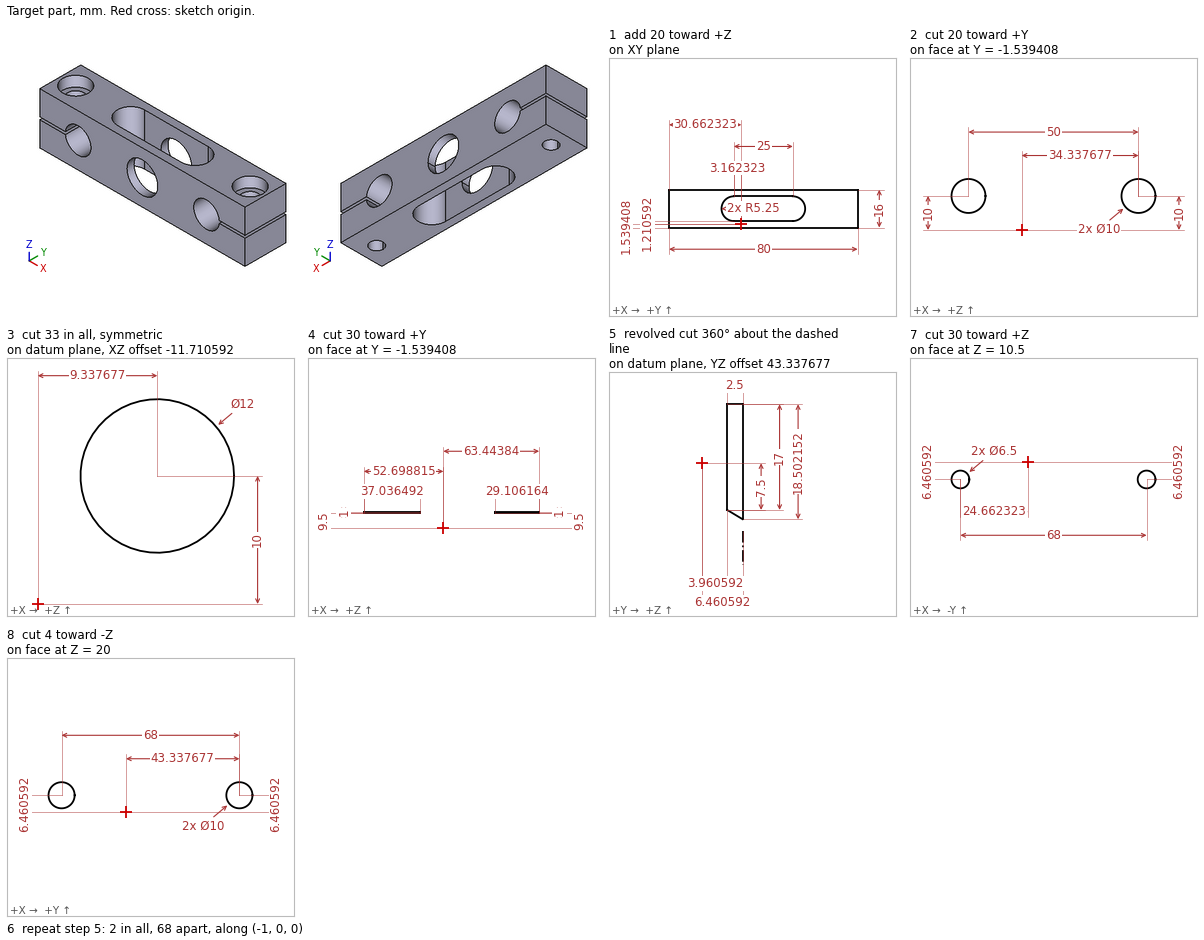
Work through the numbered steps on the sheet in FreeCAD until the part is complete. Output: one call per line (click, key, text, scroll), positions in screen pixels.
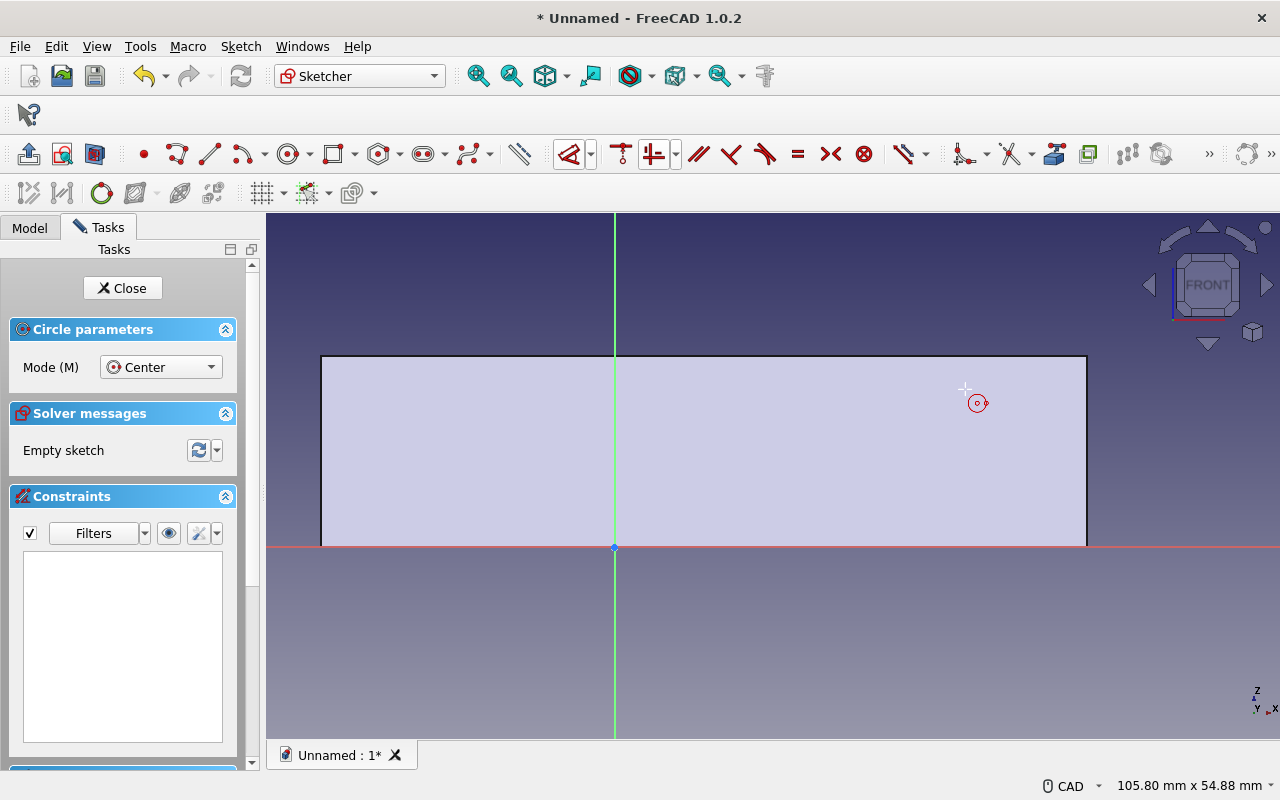
click(944, 451)
move(978, 418)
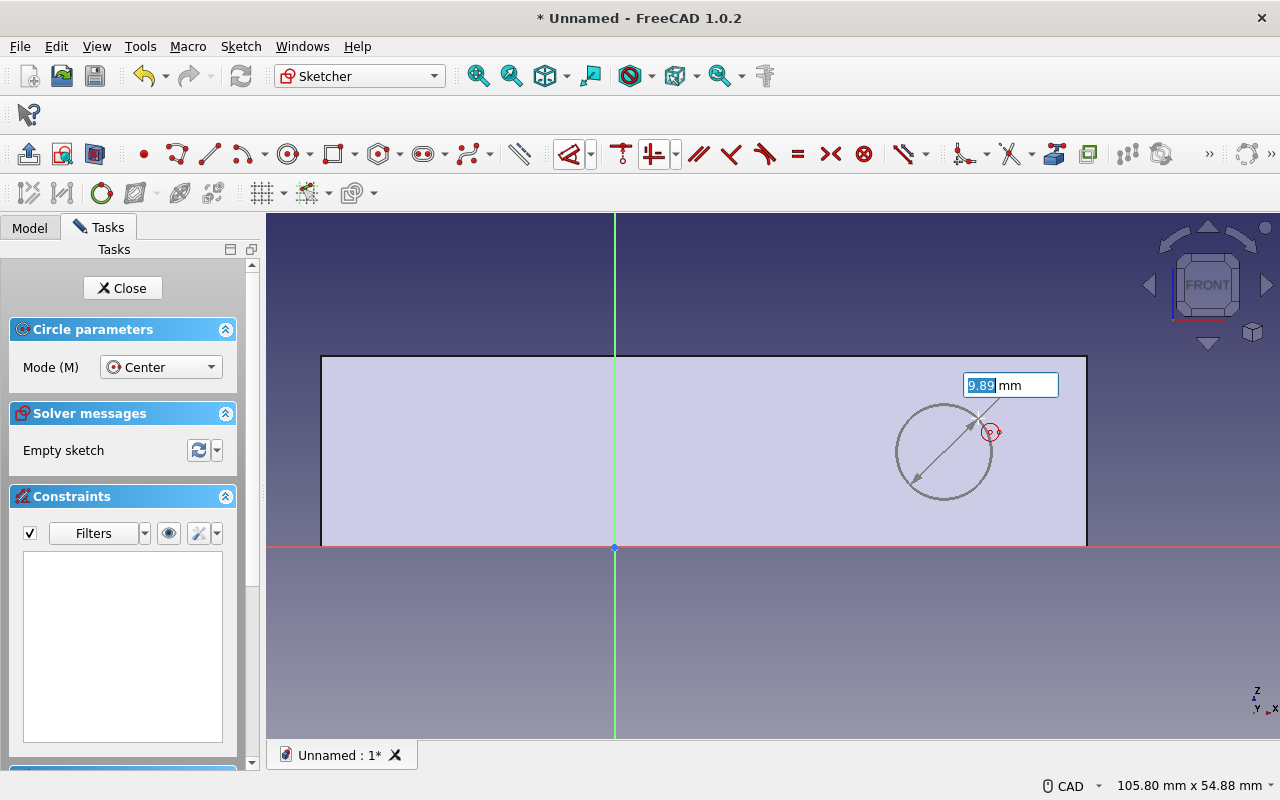
text(10)
key(Return)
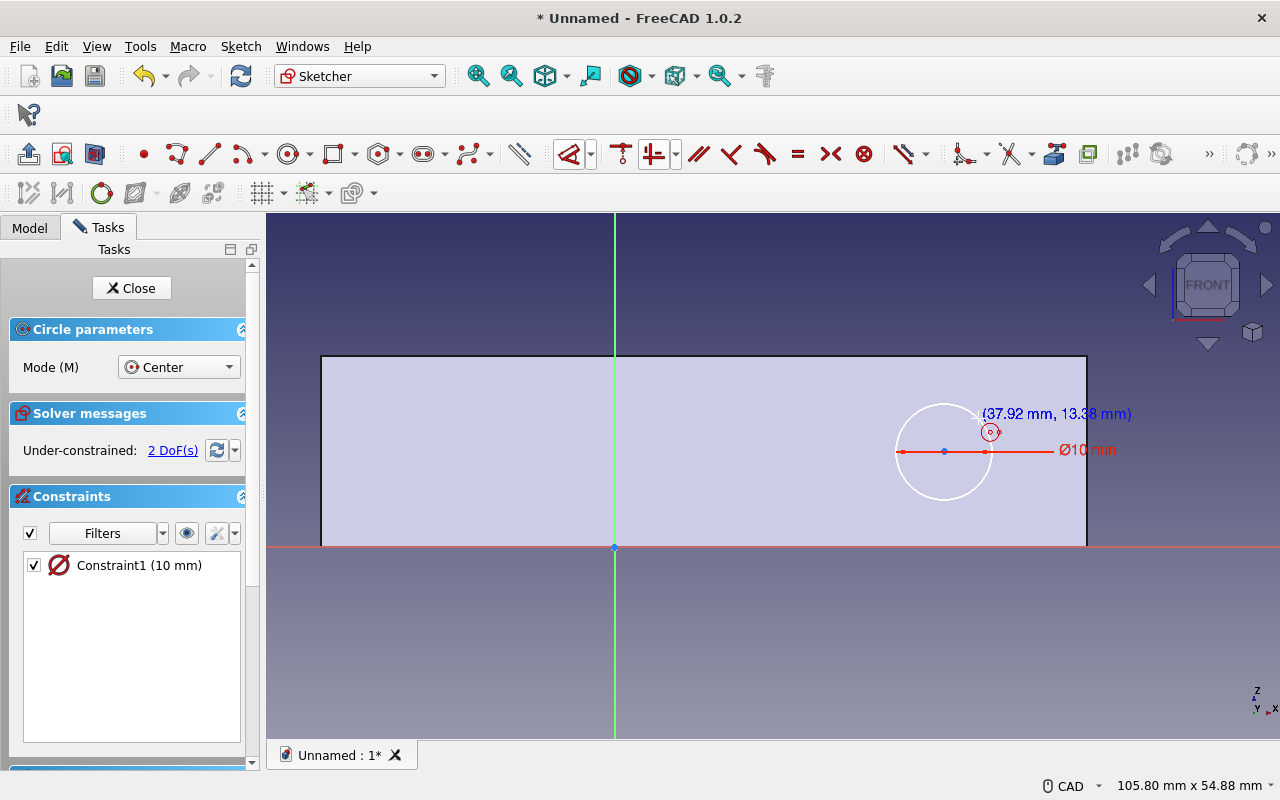
click(464, 451)
move(498, 418)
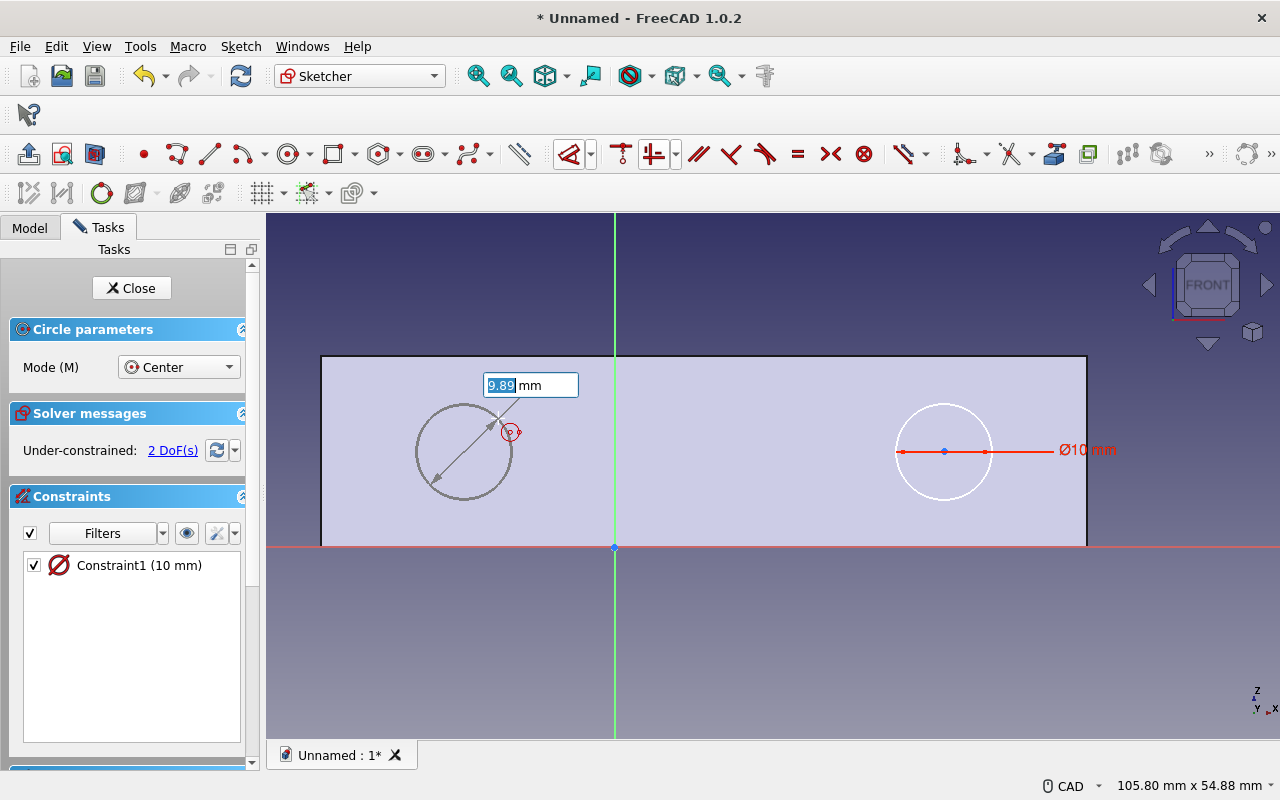
text(10)
key(Return)
key(Escape)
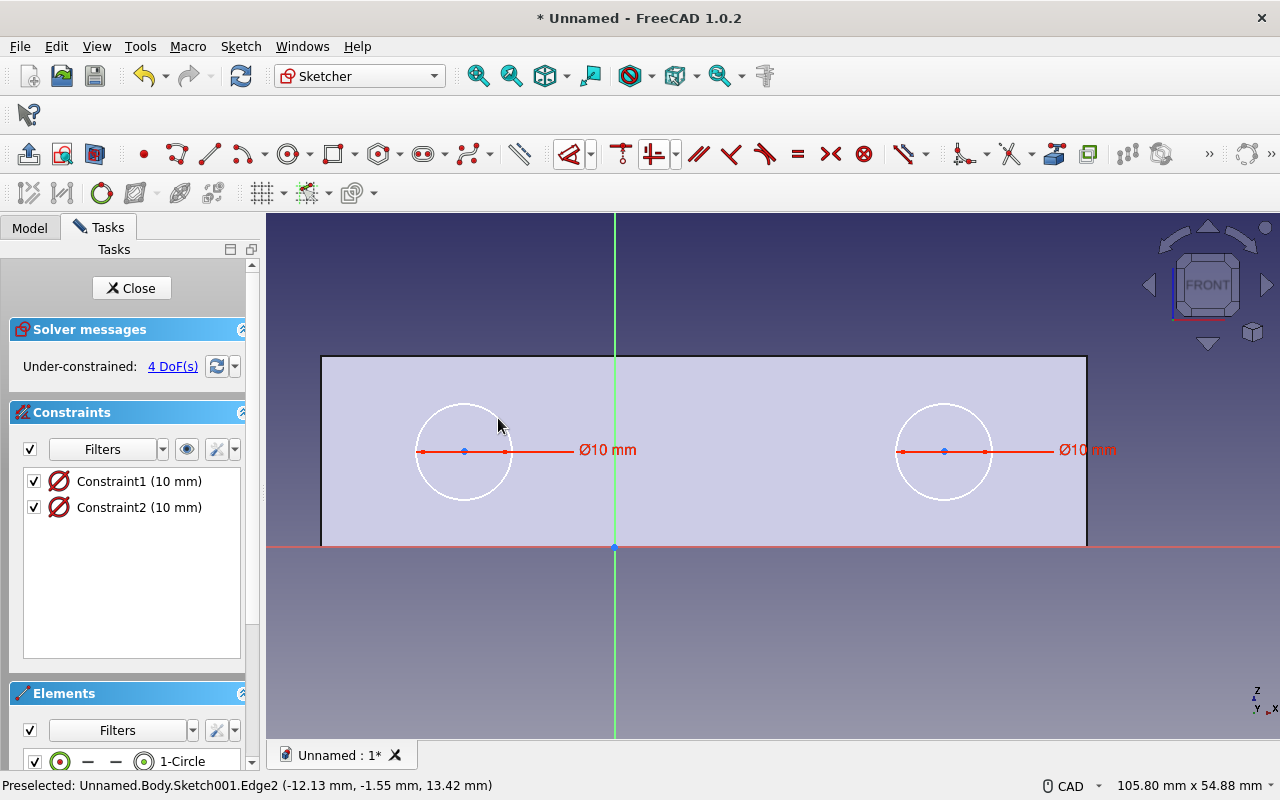
click(944, 452)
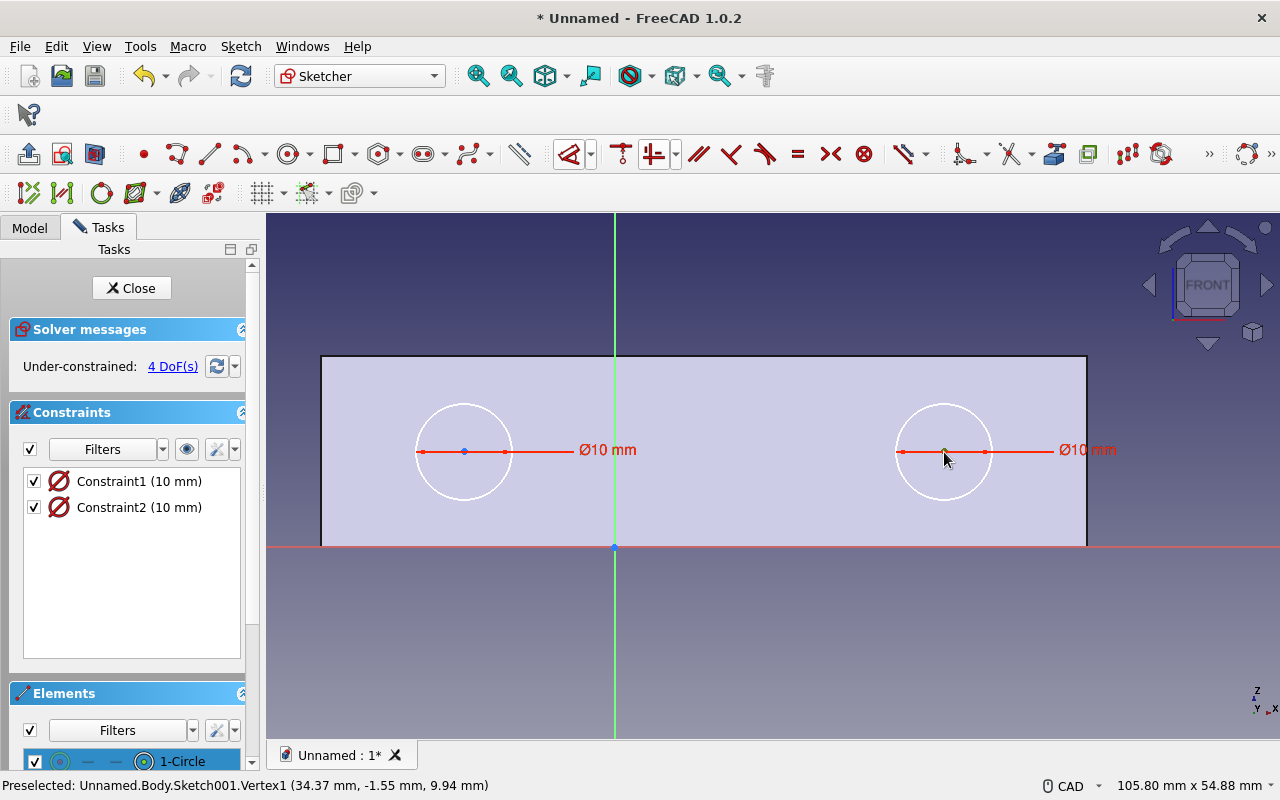
click(590, 154)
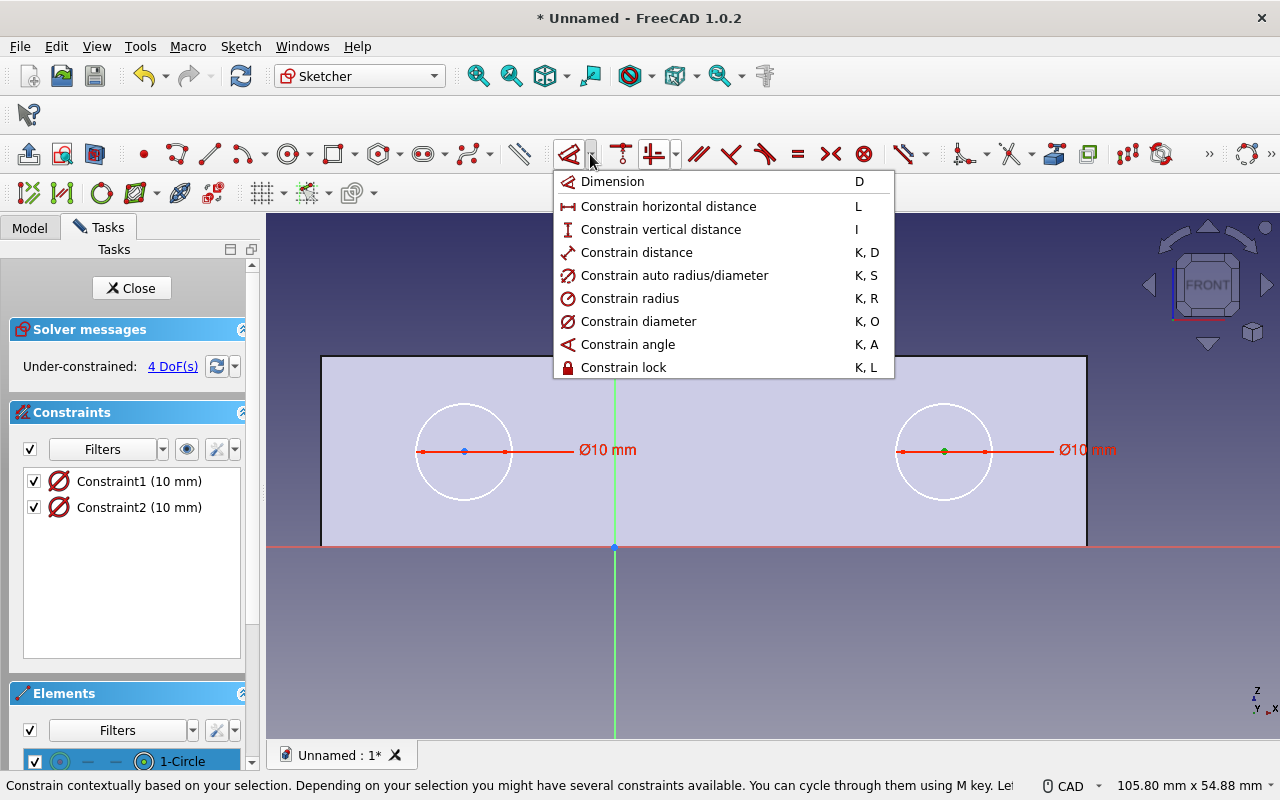
click(724, 230)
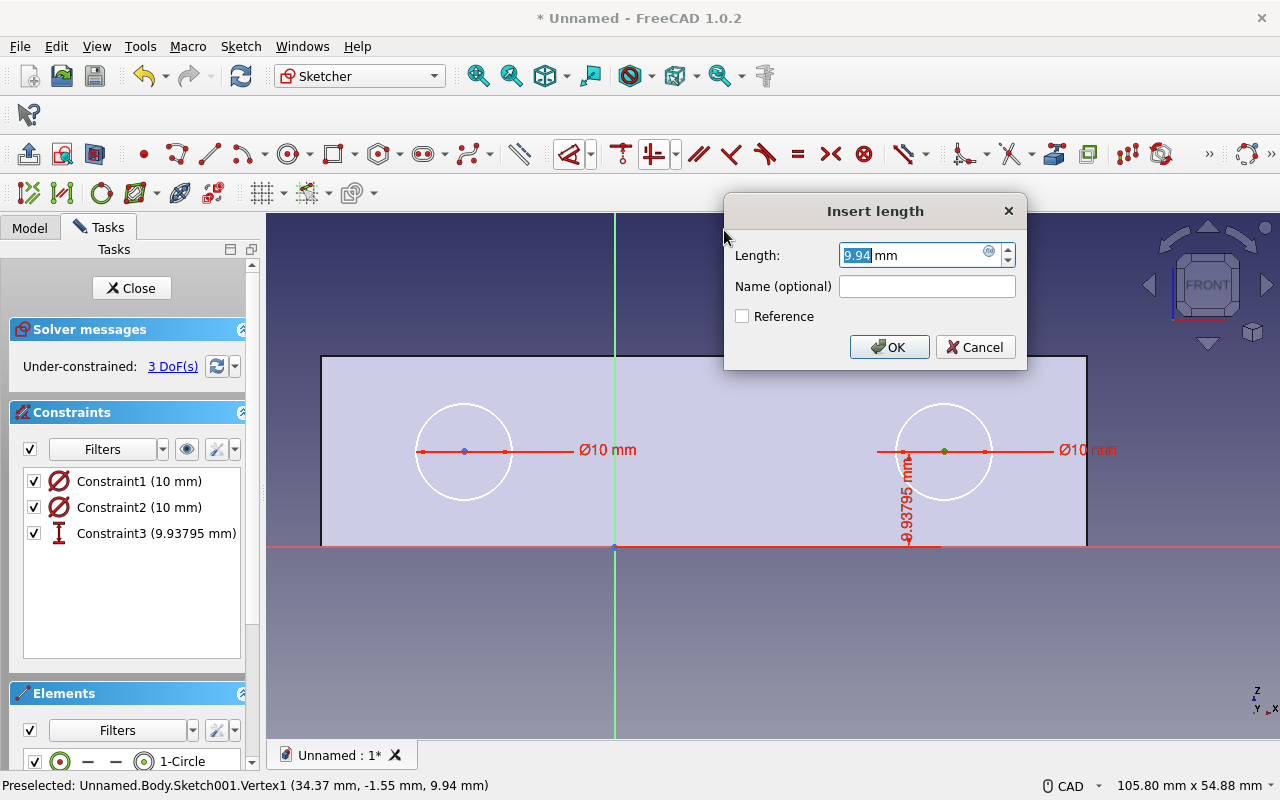
text(10)
key(Return)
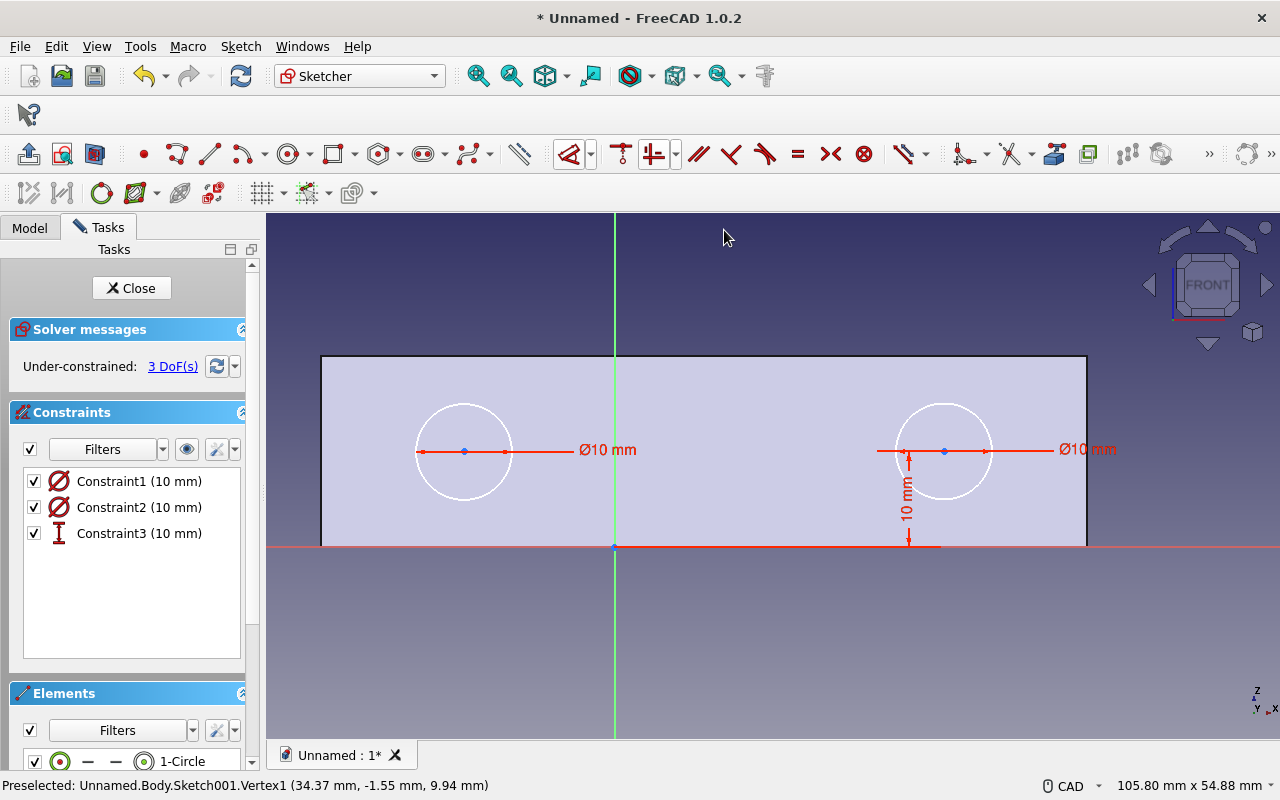
click(464, 452)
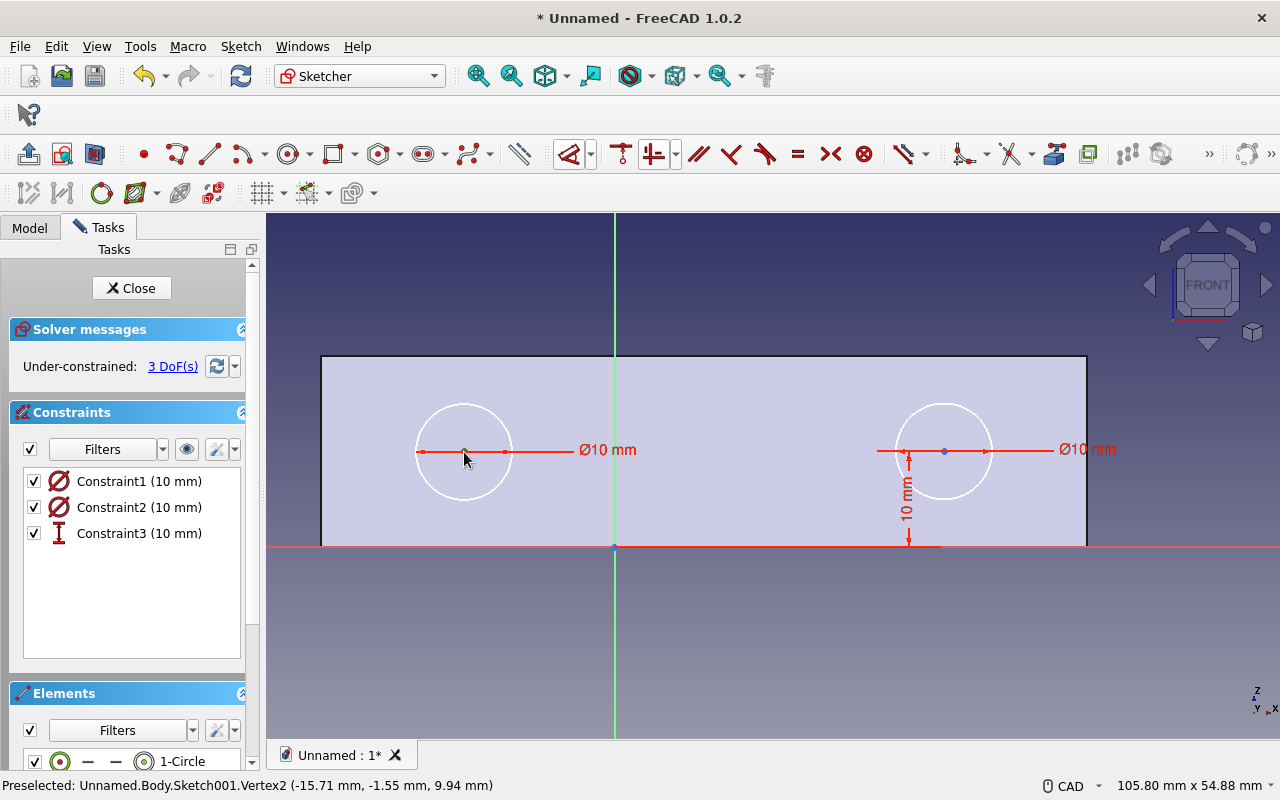
click(590, 154)